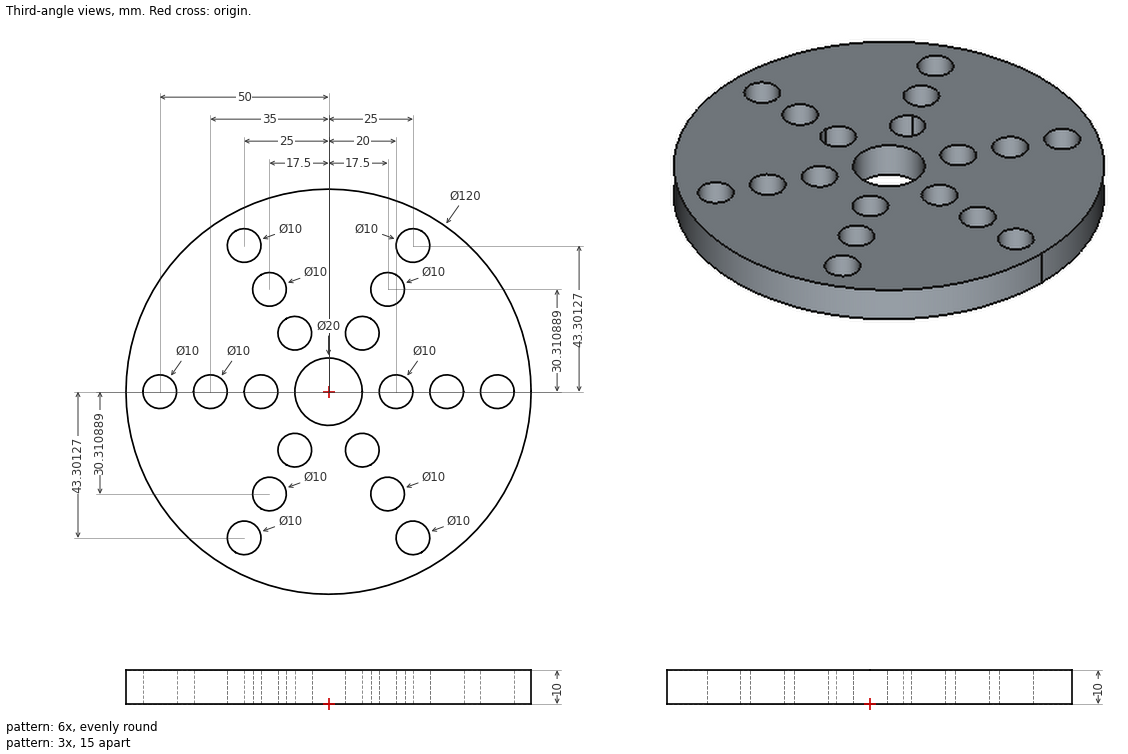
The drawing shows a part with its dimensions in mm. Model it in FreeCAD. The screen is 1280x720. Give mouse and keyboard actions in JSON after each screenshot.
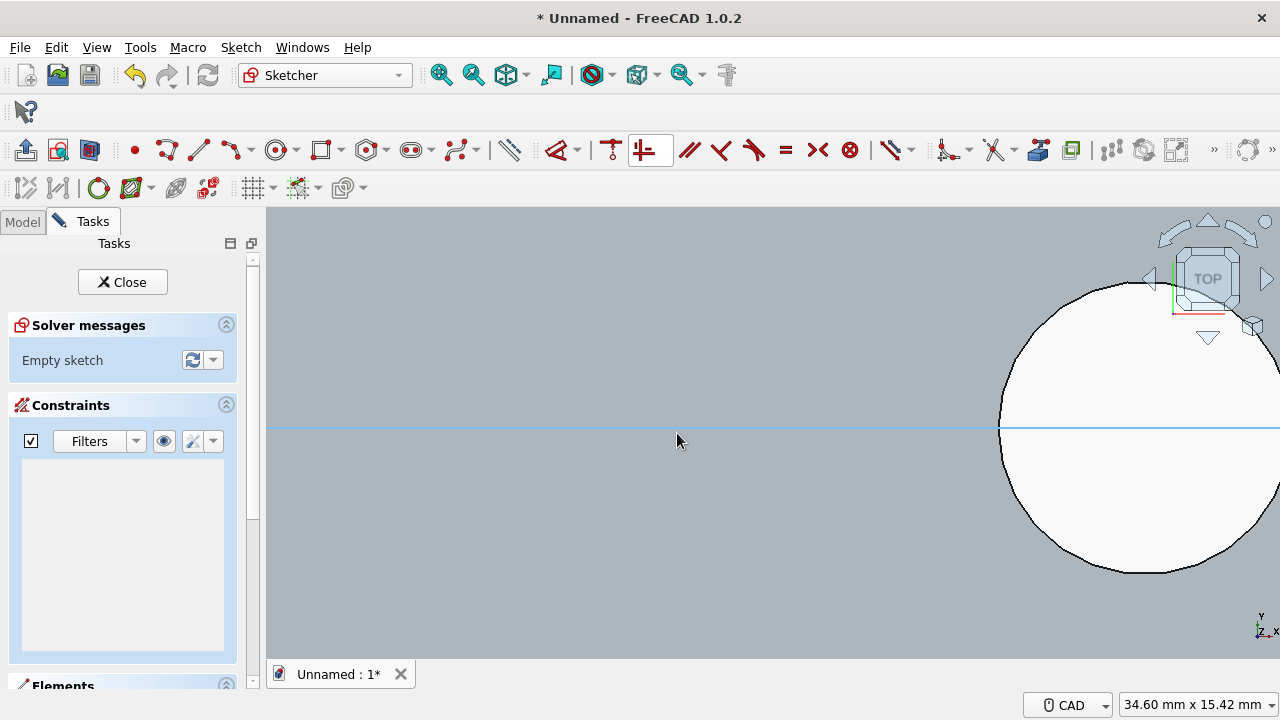
{"action": "left_click", "coordinate": [276, 150]}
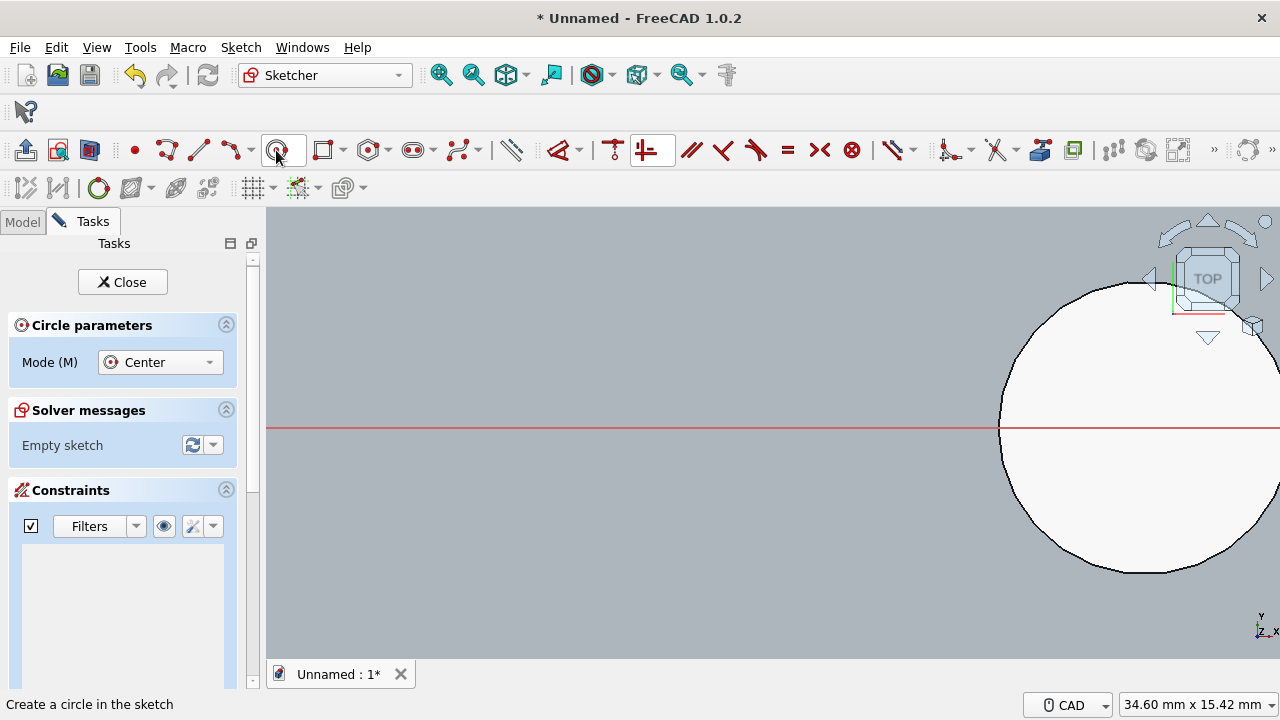
{"action": "left_click", "coordinate": [705, 428]}
{"action": "left_click", "coordinate": [809, 324]}
{"action": "key", "text": "Escape"}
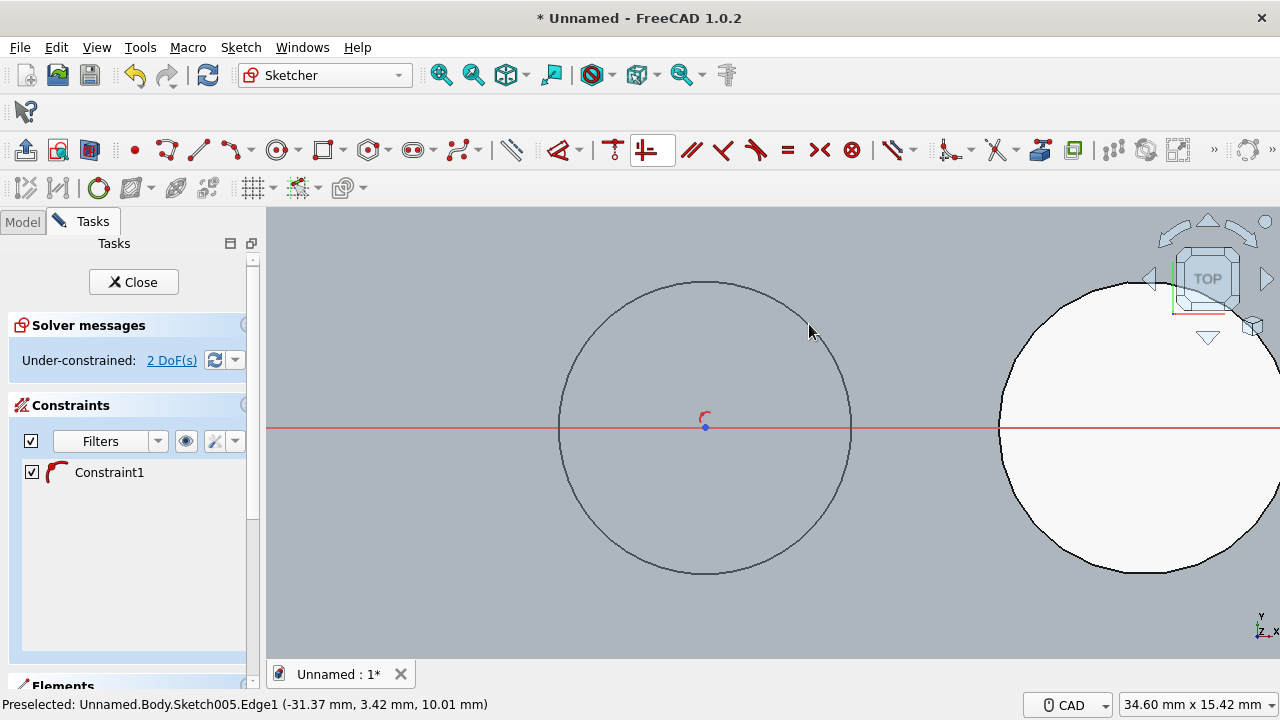
{"action": "left_click", "coordinate": [558, 150]}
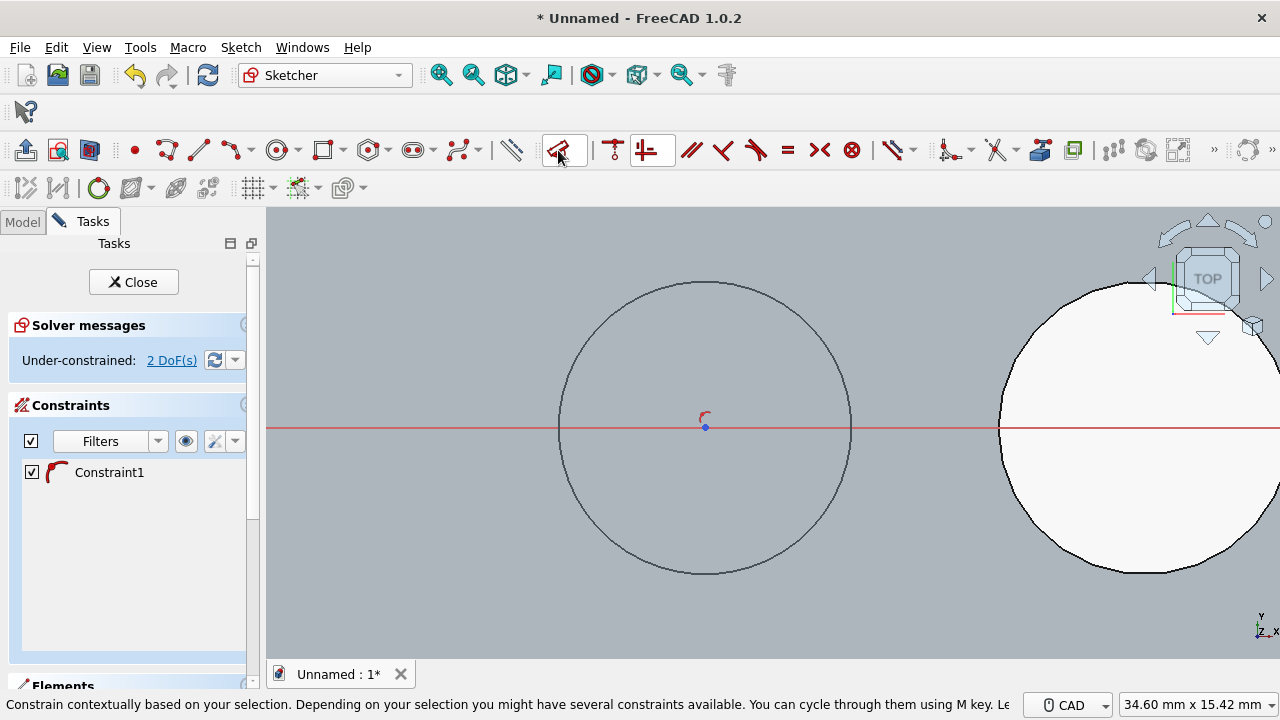
{"action": "left_click", "coordinate": [808, 324]}
{"action": "left_click", "coordinate": [831, 301]}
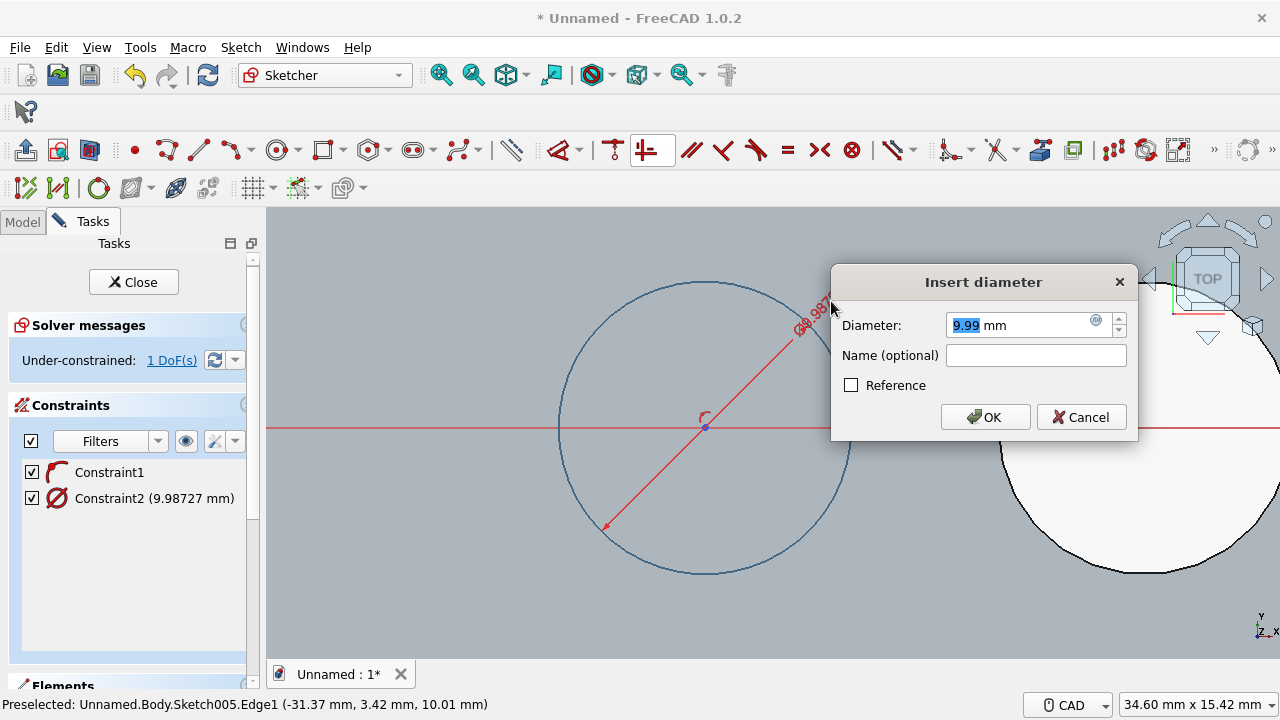
{"action": "type", "text": "10"}
{"action": "key", "text": "Return"}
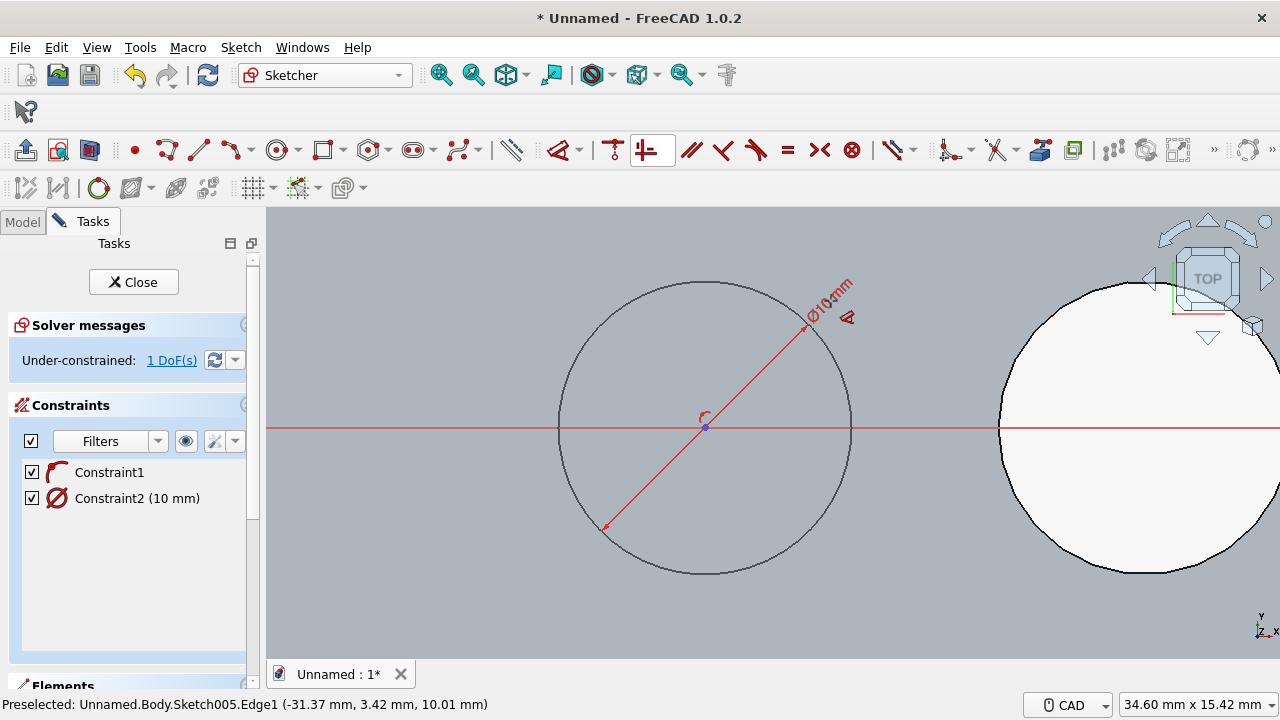
{"action": "left_click", "coordinate": [705, 428]}
{"action": "left_click", "coordinate": [910, 462]}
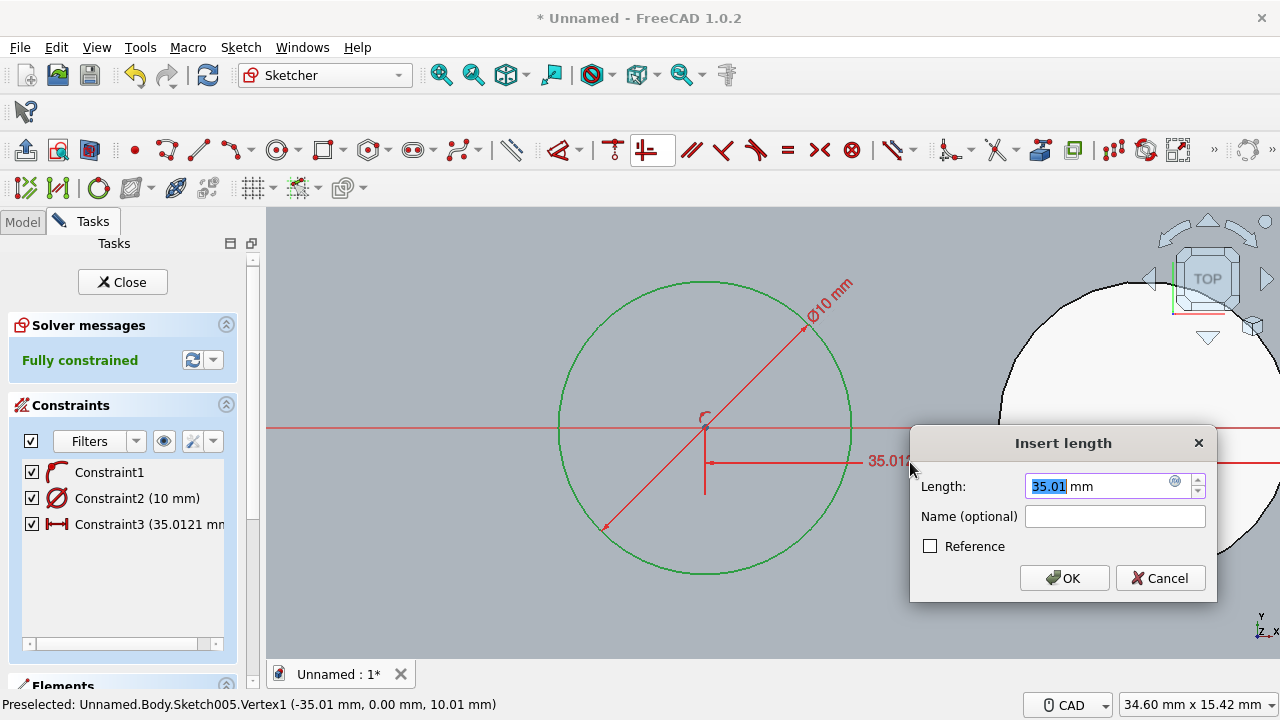
{"action": "type", "text": "35"}
{"action": "key", "text": "Return"}
{"action": "key", "text": "Escape"}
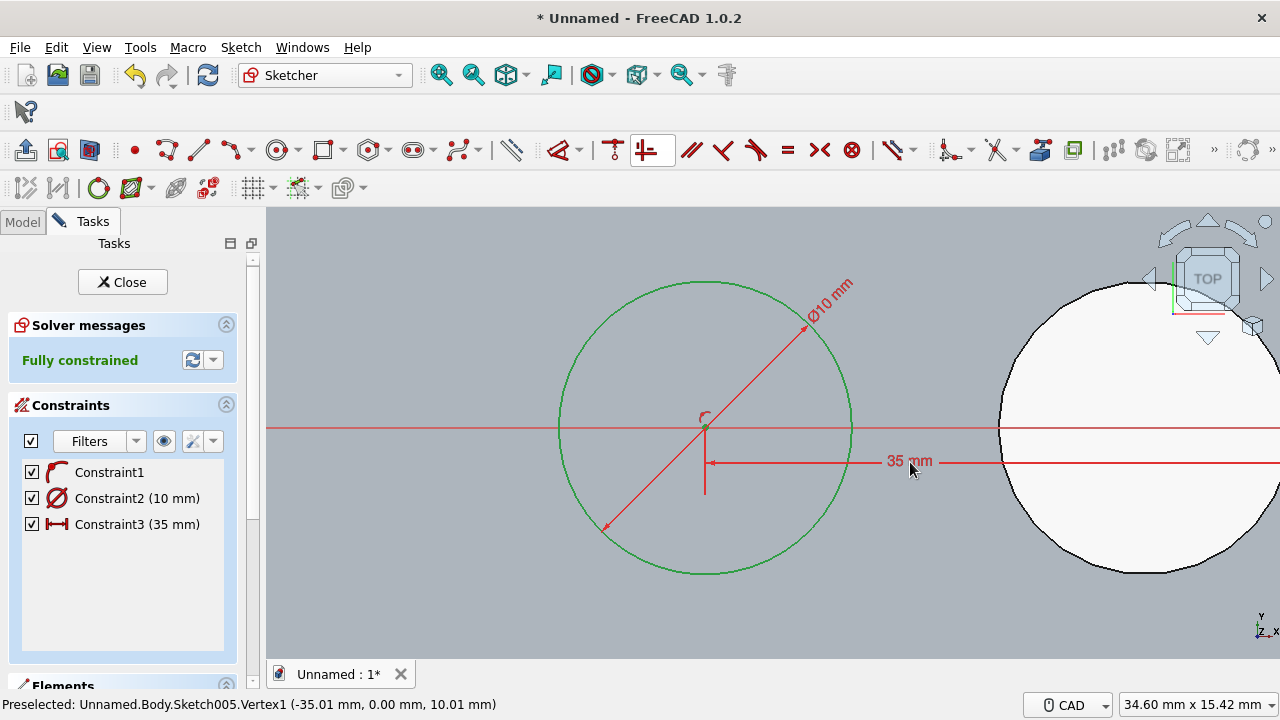
{"action": "left_click", "coordinate": [123, 282]}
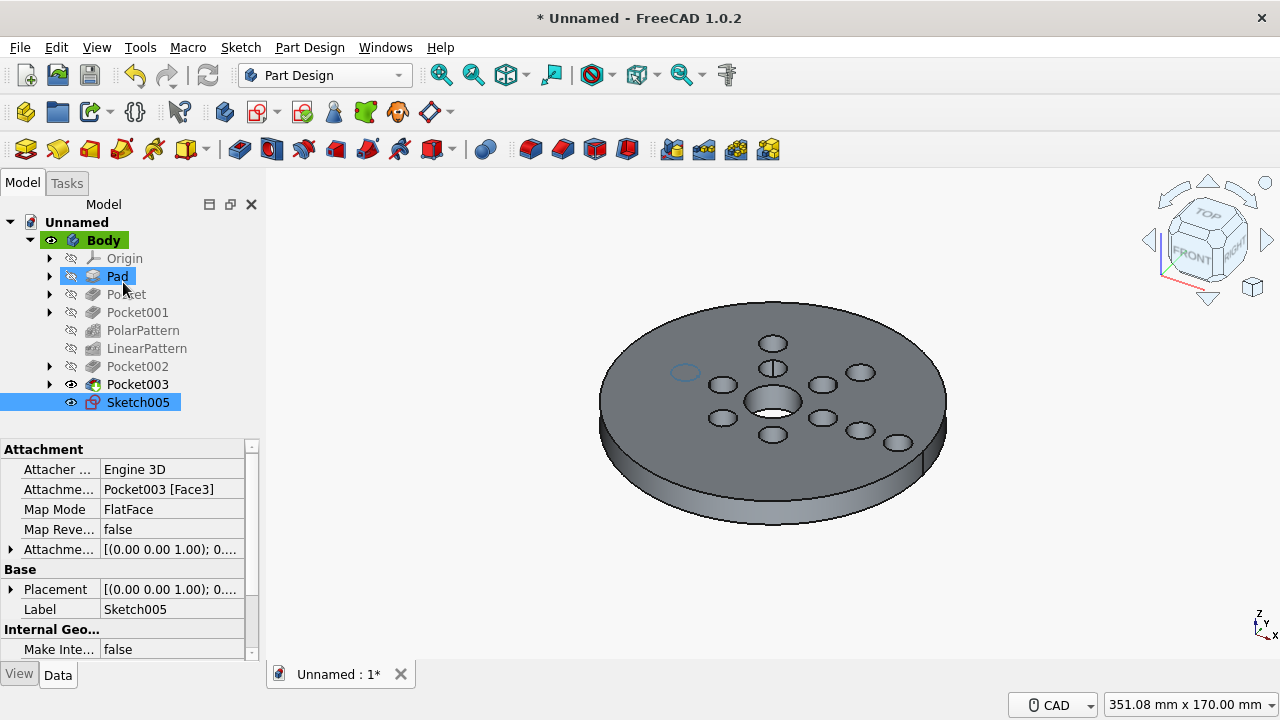
{"action": "left_click", "coordinate": [240, 150]}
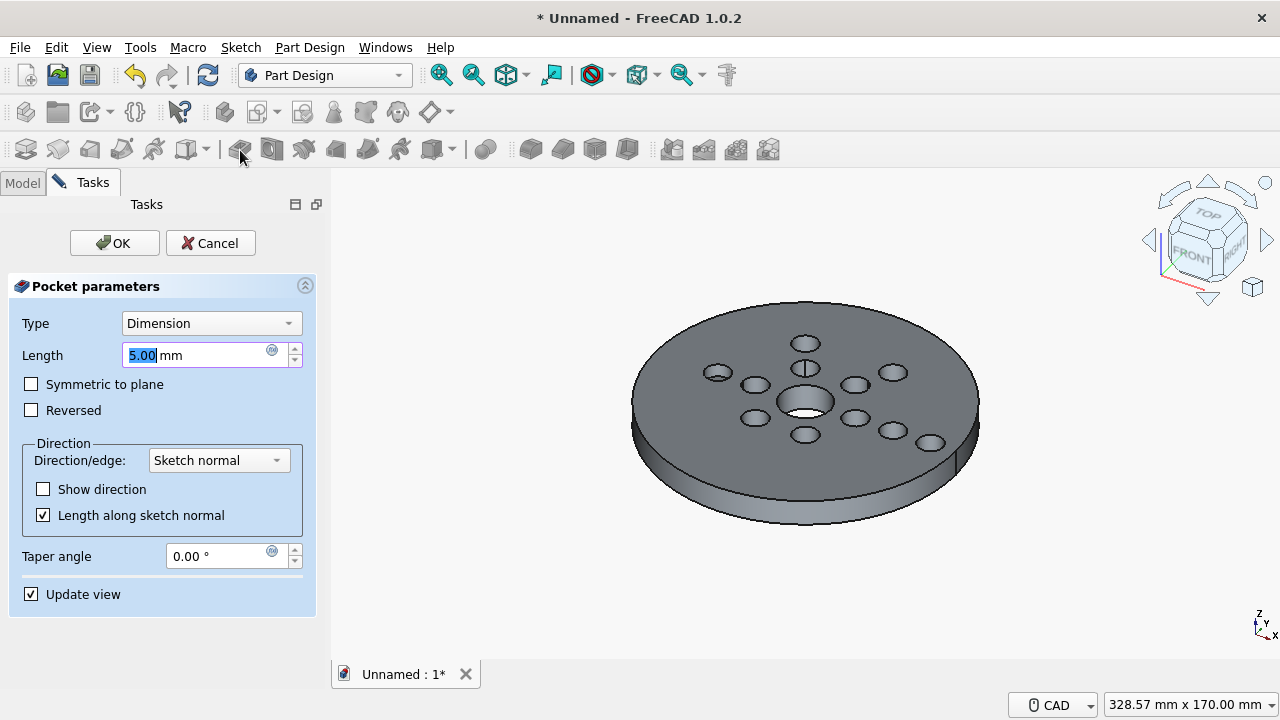
{"action": "type", "text": "10"}
{"action": "key", "text": "Tab"}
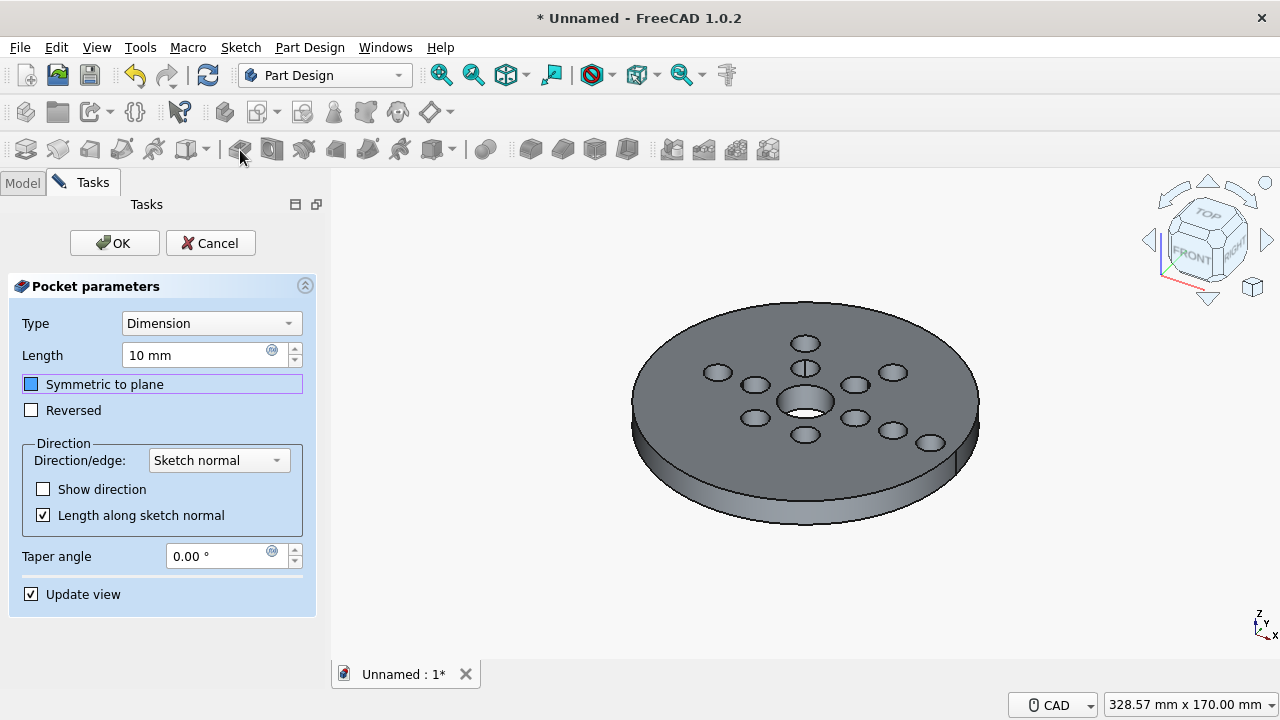
{"action": "left_click", "coordinate": [115, 243]}